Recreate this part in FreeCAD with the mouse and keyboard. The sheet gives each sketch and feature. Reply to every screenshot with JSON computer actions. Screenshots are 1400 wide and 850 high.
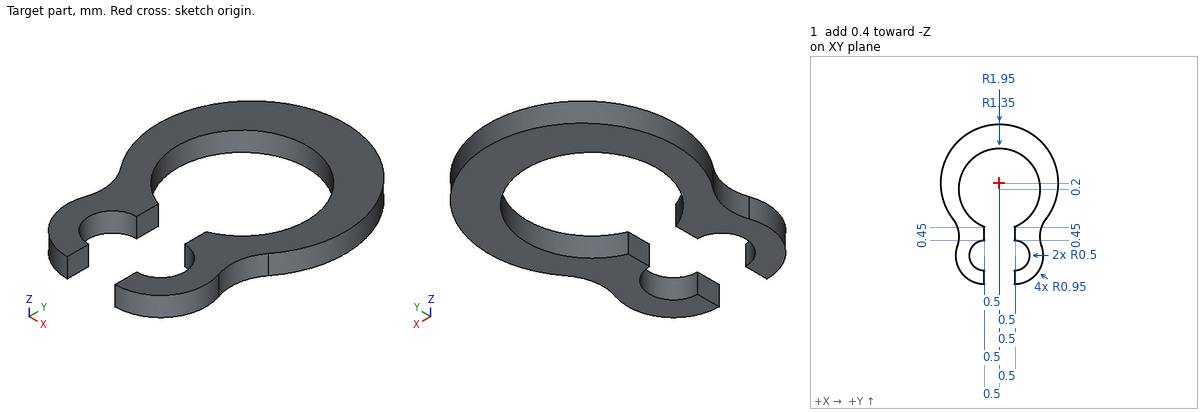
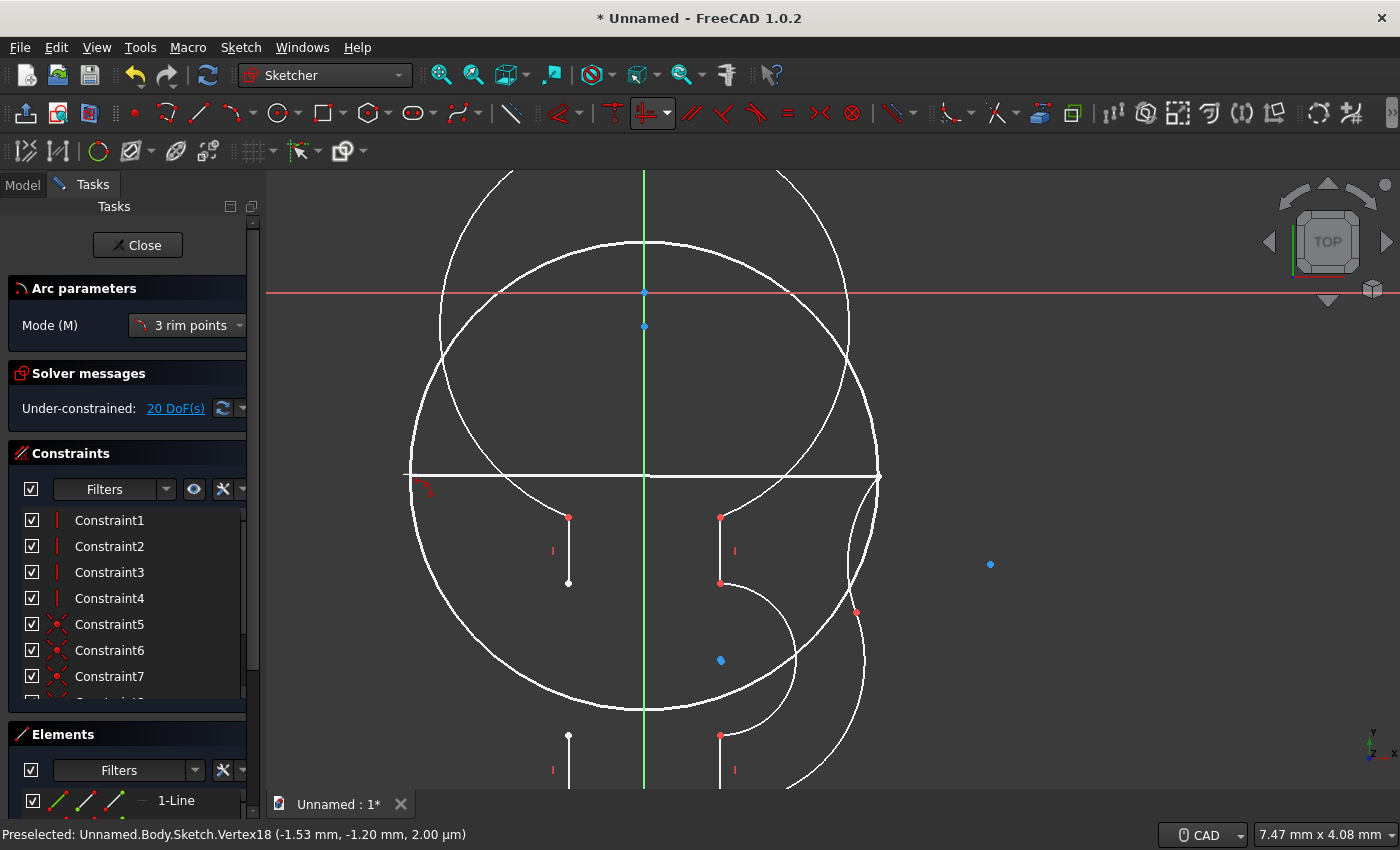
{"action": "scroll", "coordinate": [863, 545], "scroll_direction": "down", "scroll_amount": 4}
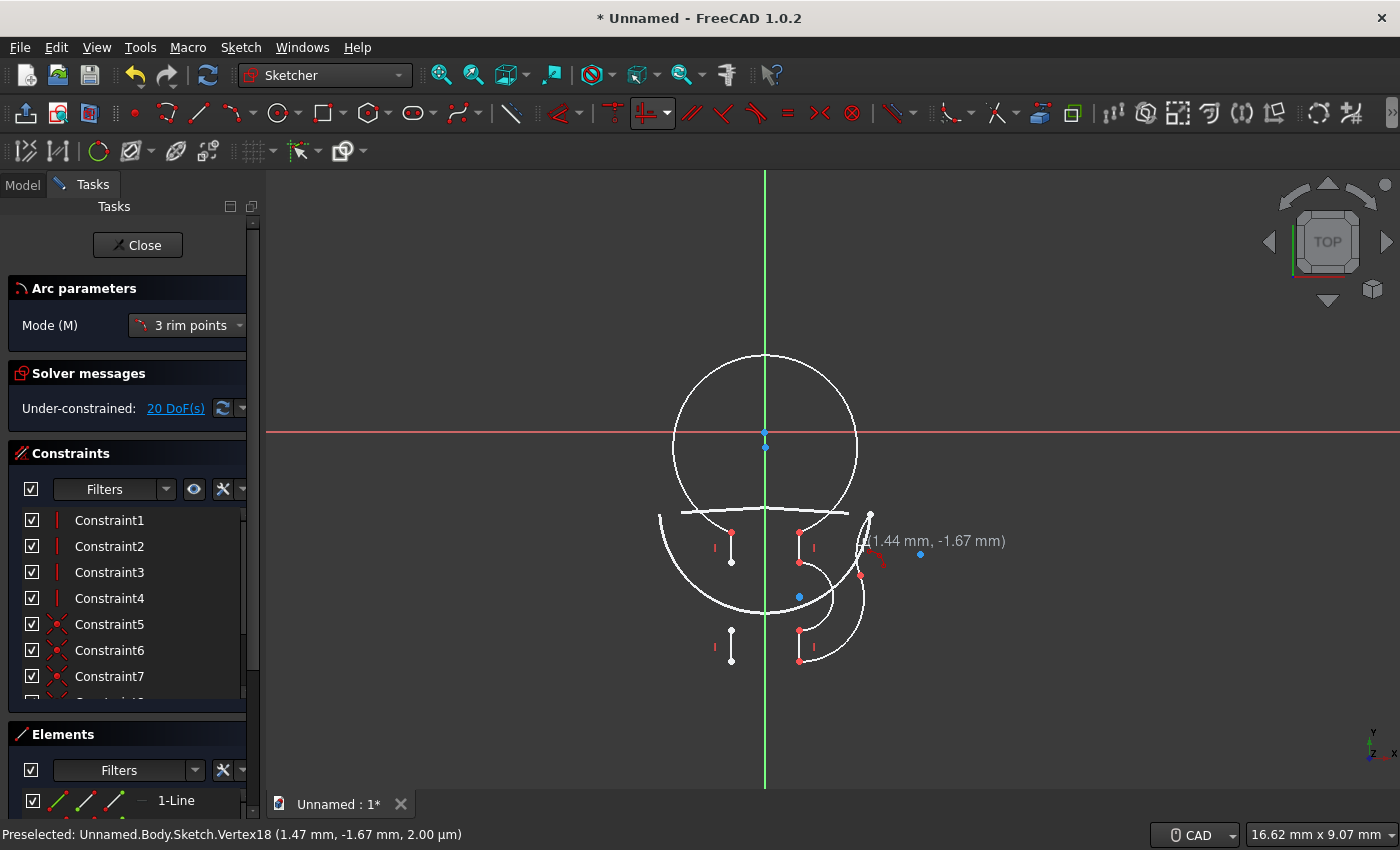
{"action": "left_click", "coordinate": [822, 312]}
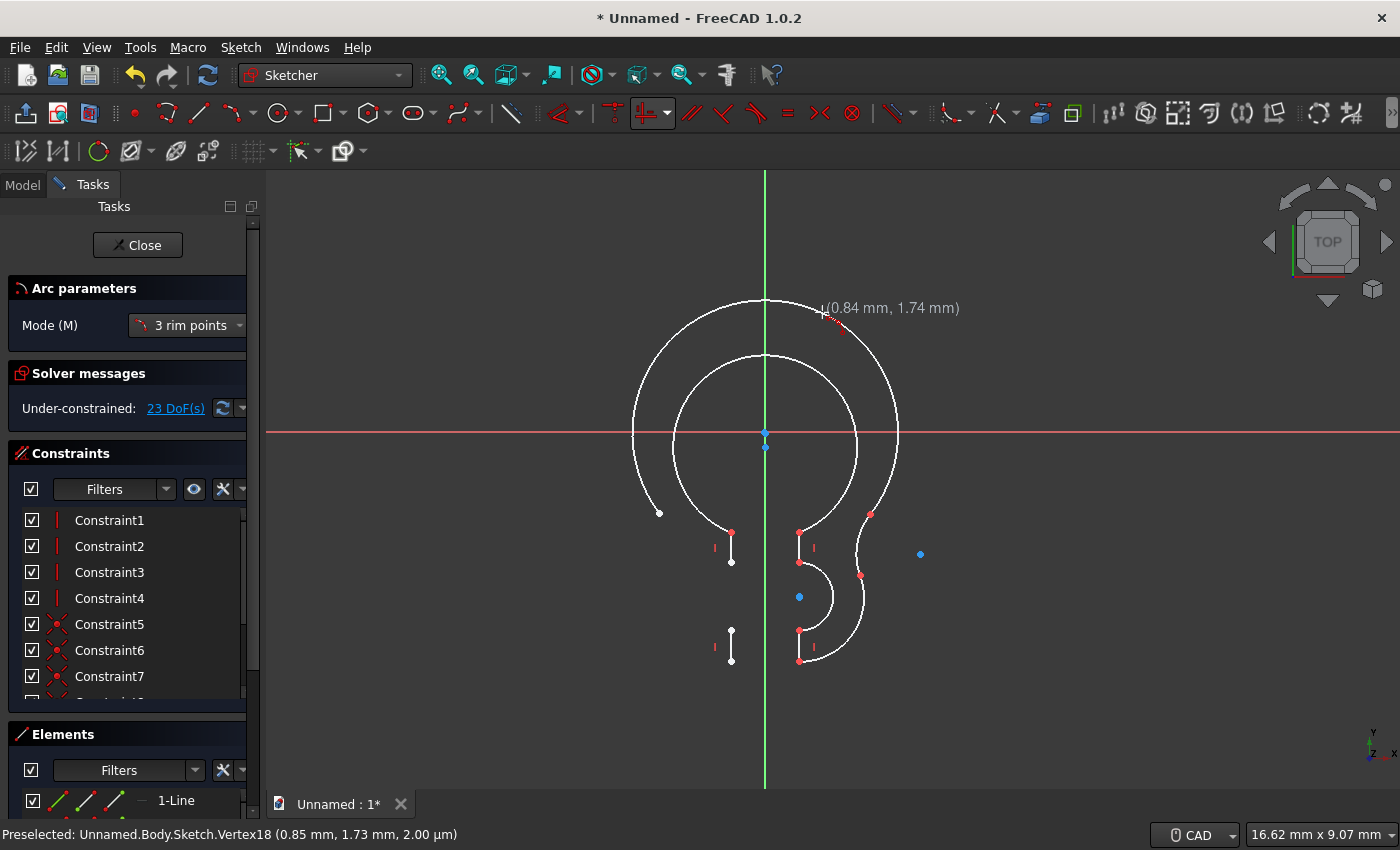
{"action": "left_click", "coordinate": [660, 514]}
{"action": "left_click", "coordinate": [670, 575]}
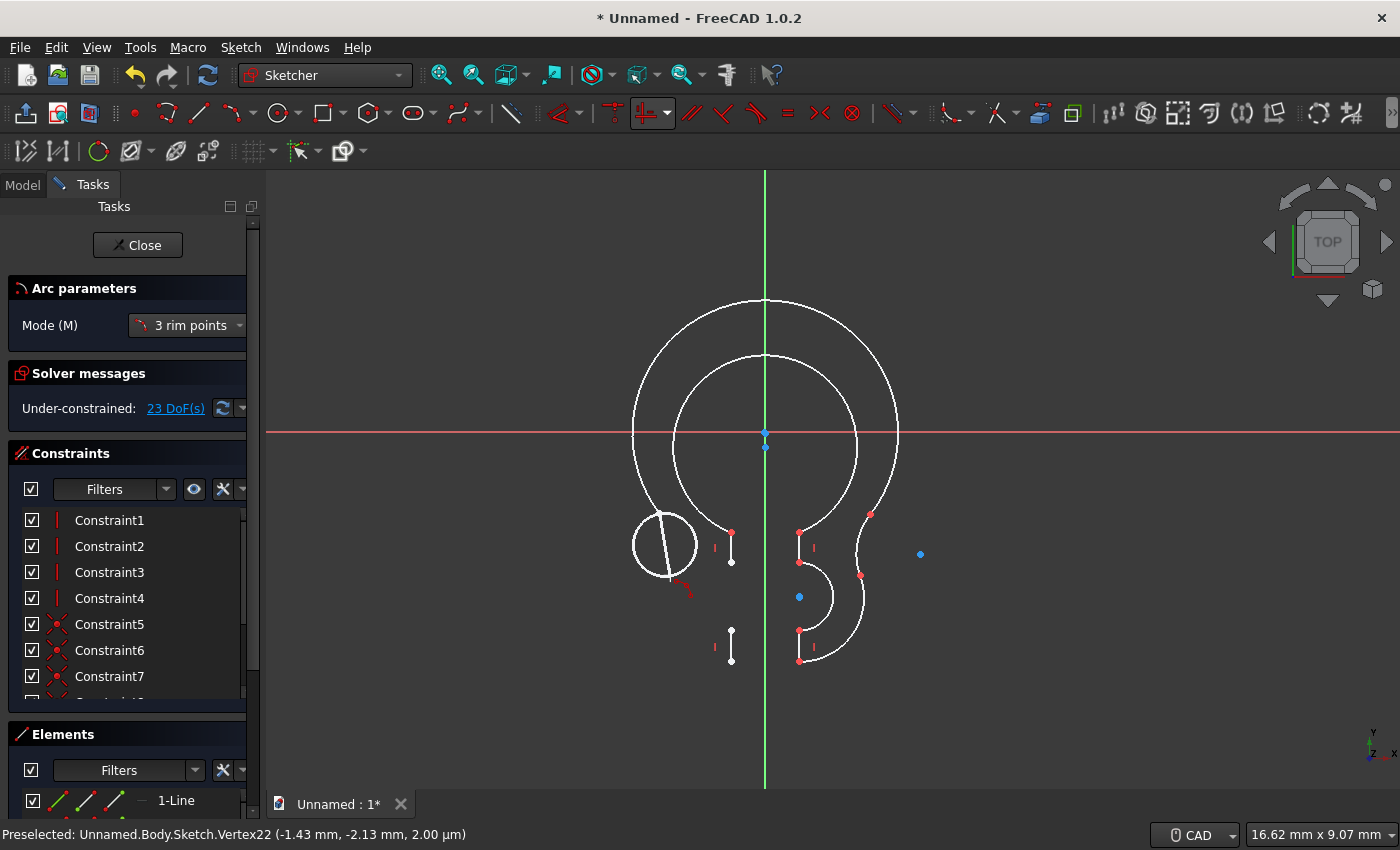
{"action": "scroll", "coordinate": [672, 543], "scroll_direction": "up", "scroll_amount": 4}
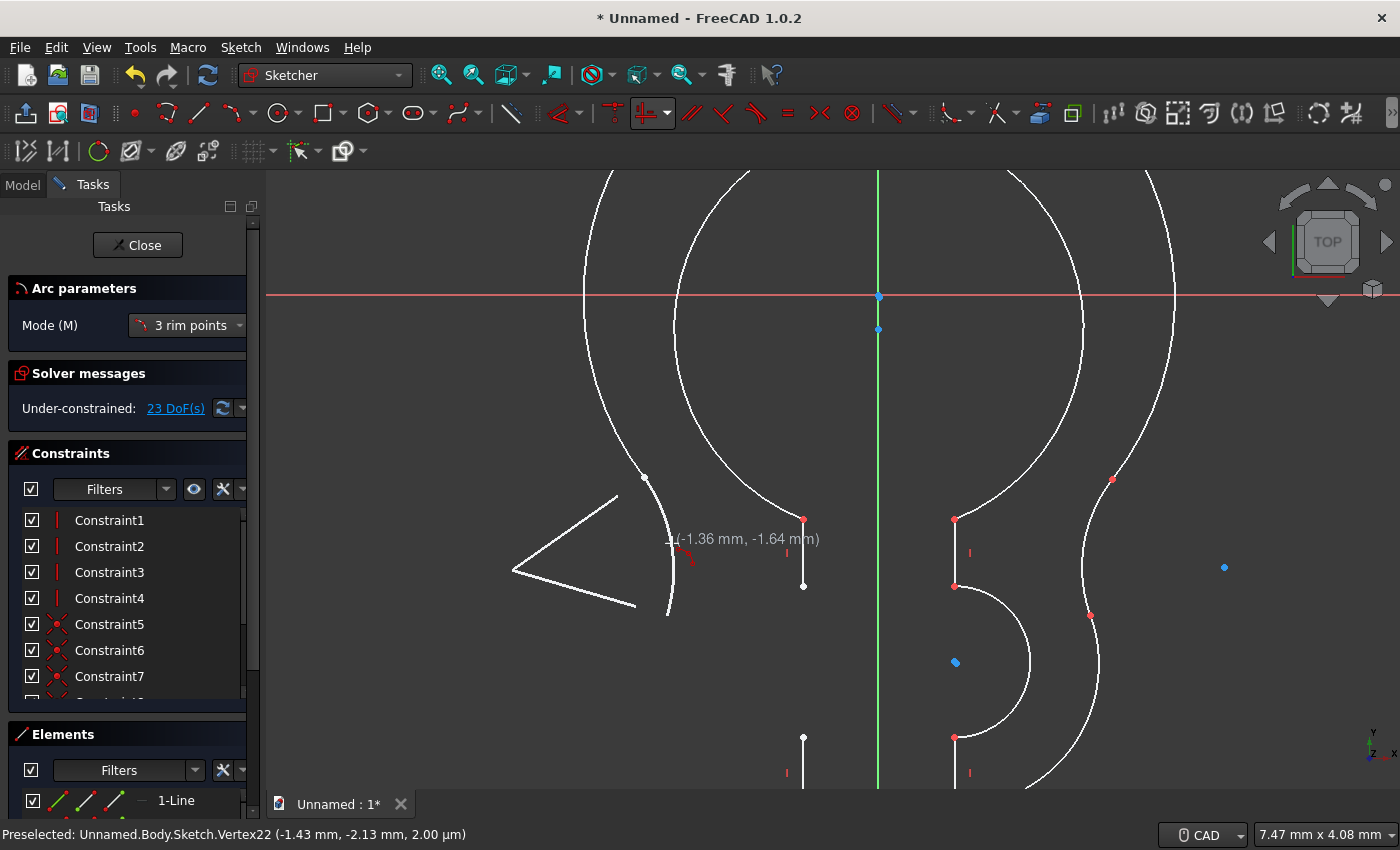
{"action": "left_click", "coordinate": [673, 542]}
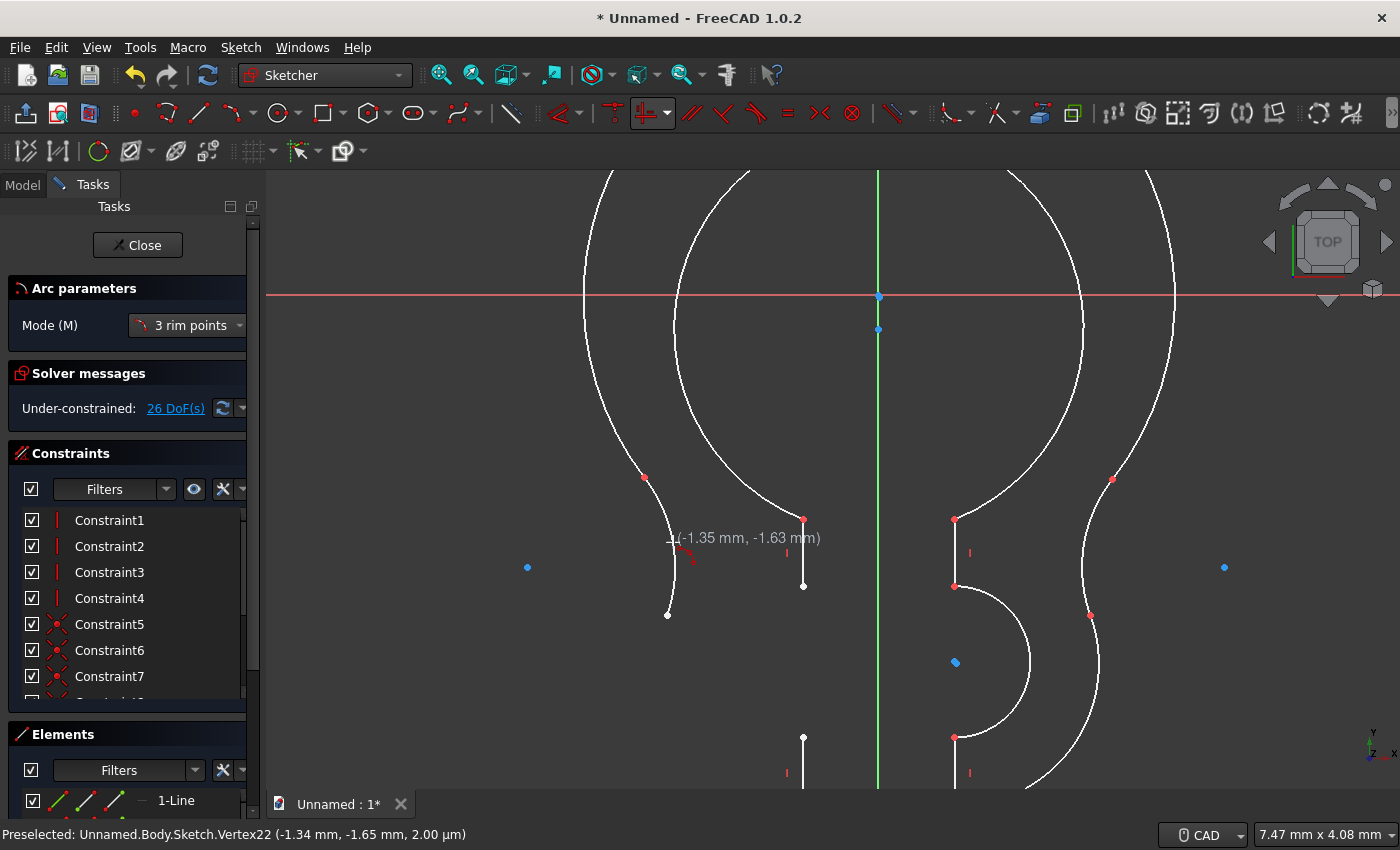
{"action": "left_click", "coordinate": [667, 616]}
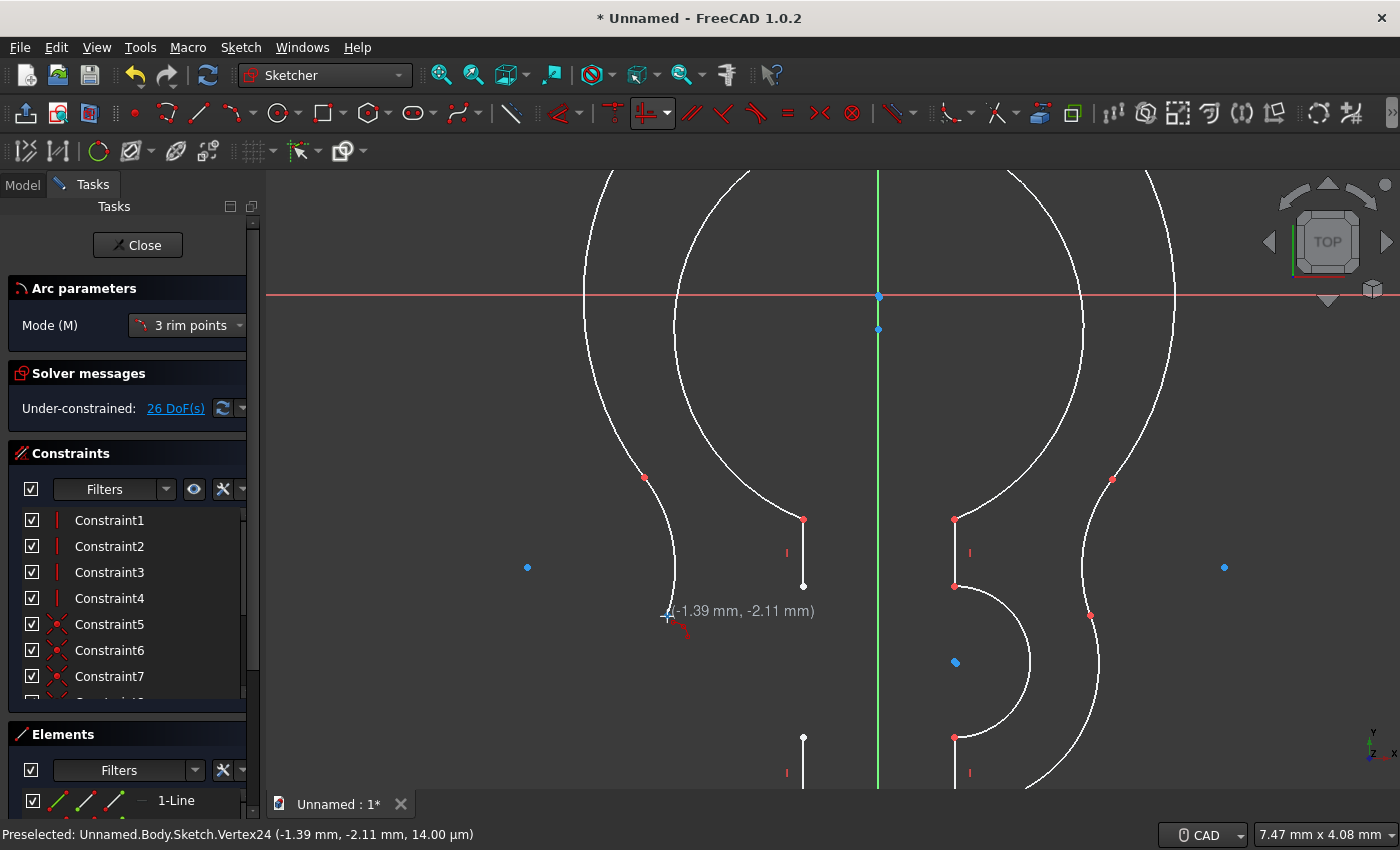
{"action": "scroll", "coordinate": [672, 543], "scroll_direction": "down", "scroll_amount": 4}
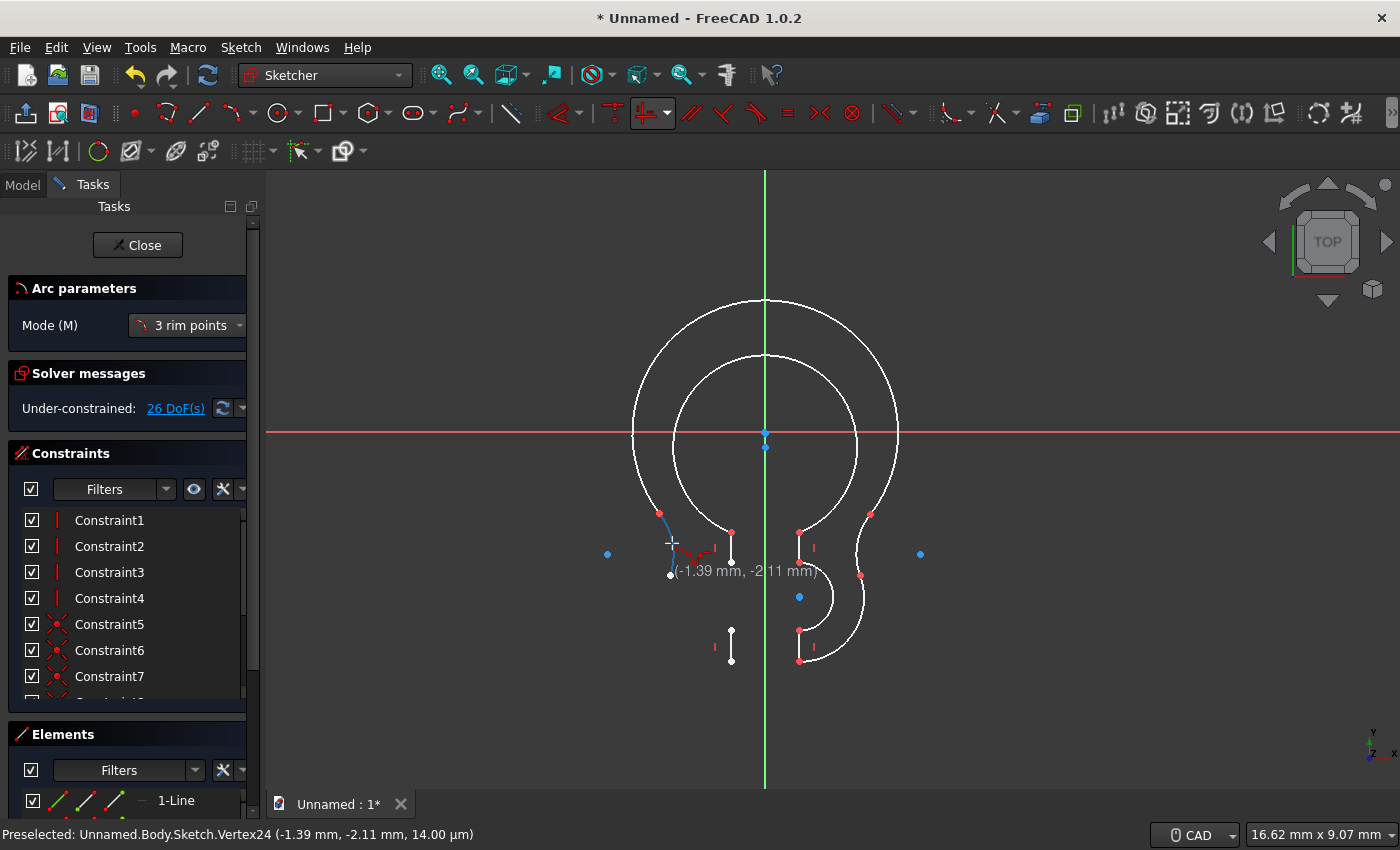
{"action": "left_click", "coordinate": [731, 662]}
{"action": "left_click", "coordinate": [678, 634]}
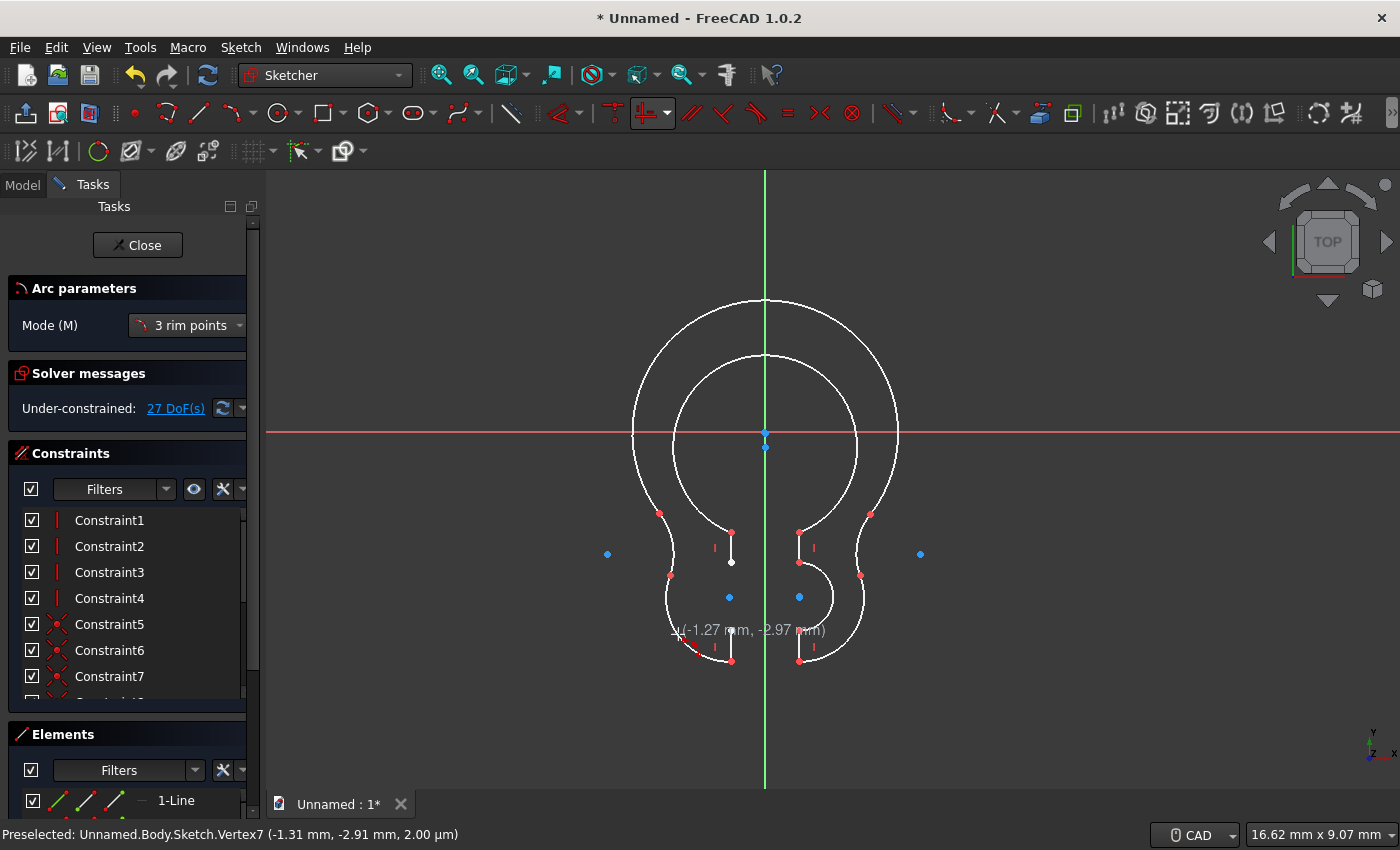
{"action": "left_click", "coordinate": [731, 631]}
{"action": "left_click", "coordinate": [731, 563]}
{"action": "left_click", "coordinate": [697, 596]}
{"action": "key", "text": "Escape"}